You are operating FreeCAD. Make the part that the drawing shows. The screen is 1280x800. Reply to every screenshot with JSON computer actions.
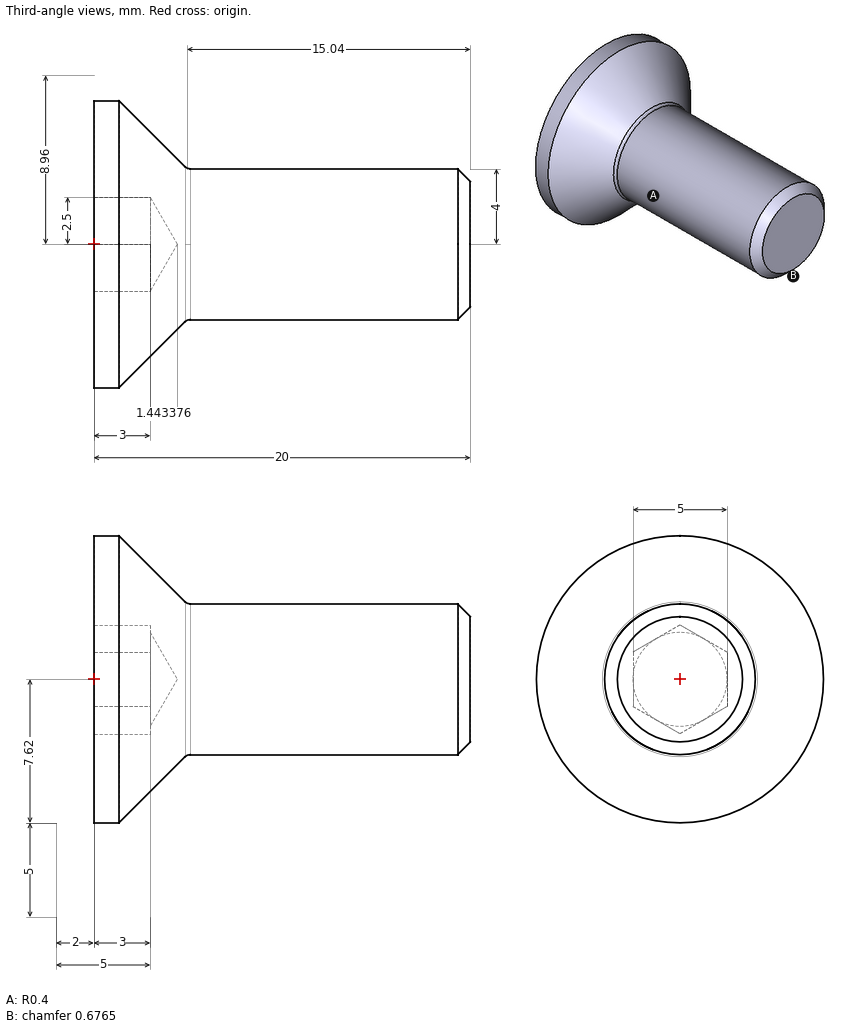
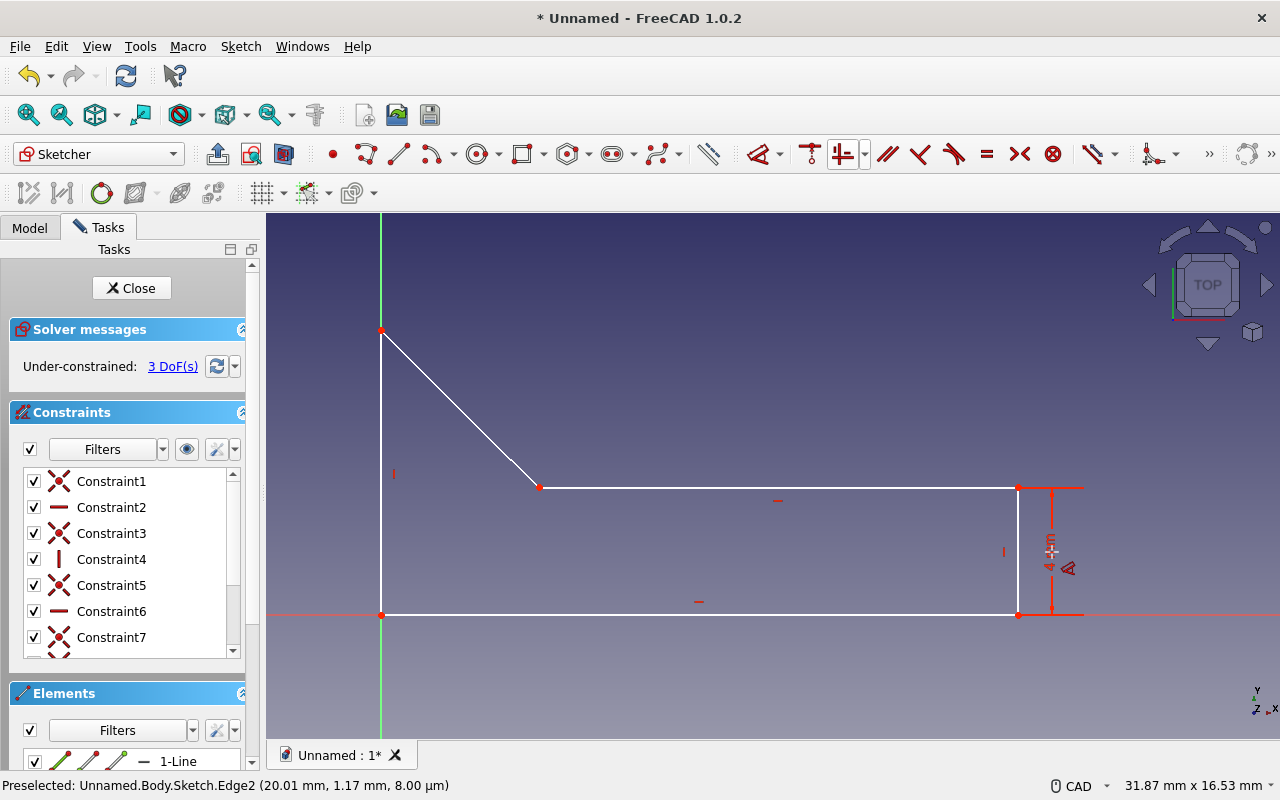
{"action": "left_click", "coordinate": [572, 615]}
{"action": "left_click", "coordinate": [700, 649]}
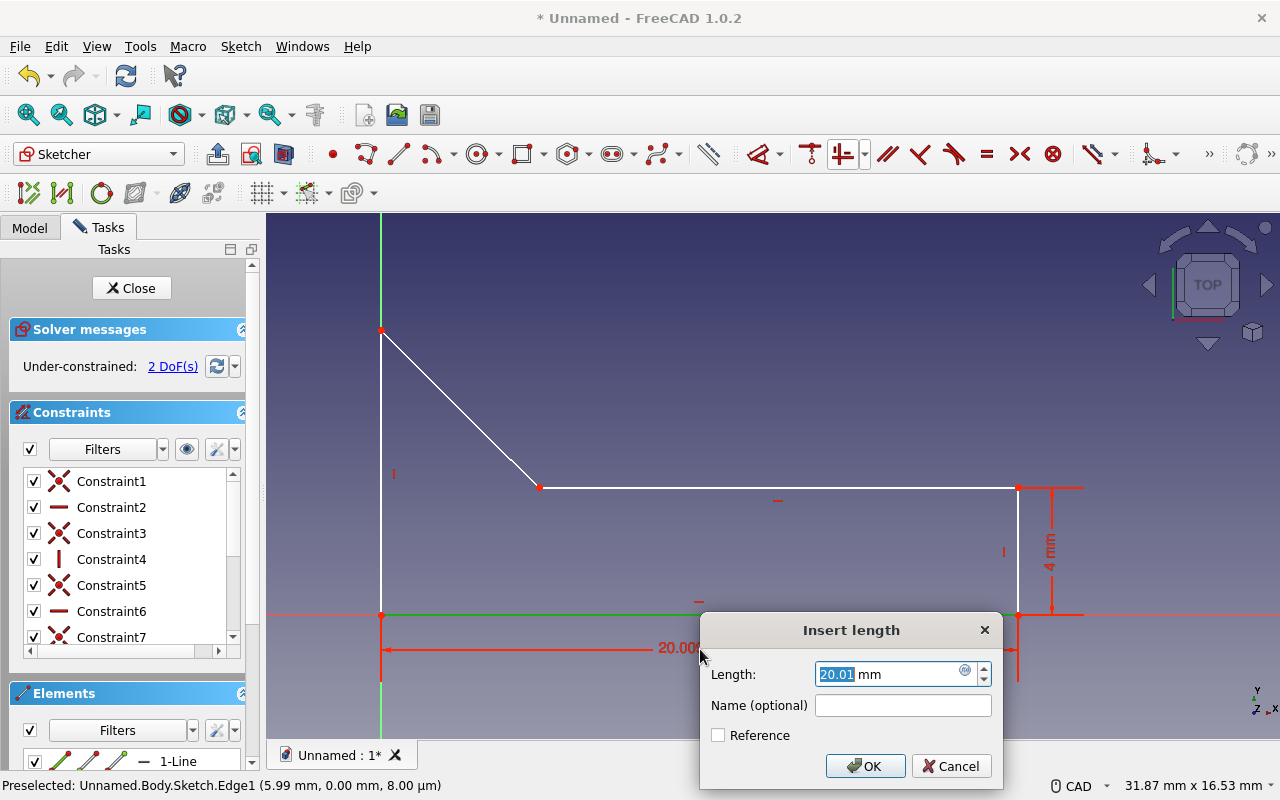
{"action": "type", "text": "20"}
{"action": "key", "text": "Return"}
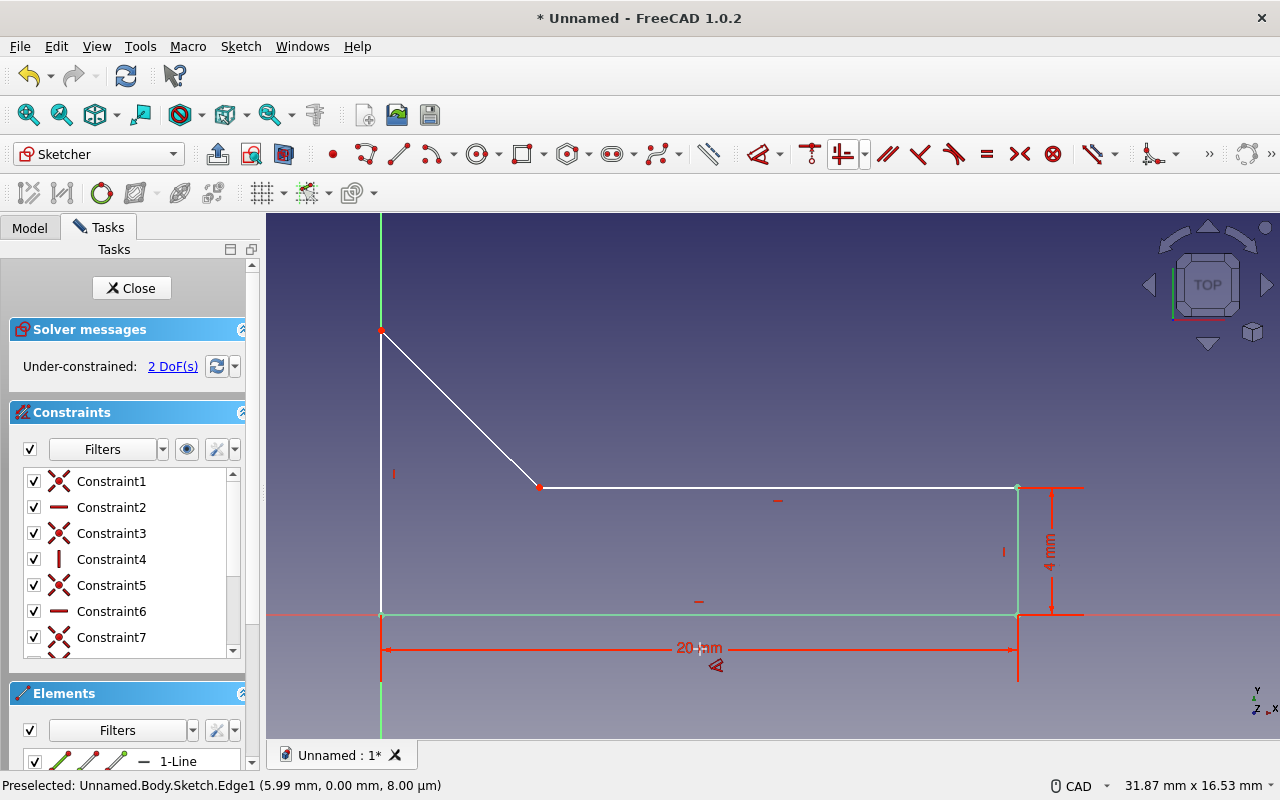
{"action": "left_click", "coordinate": [381, 416]}
{"action": "left_click", "coordinate": [347, 473]}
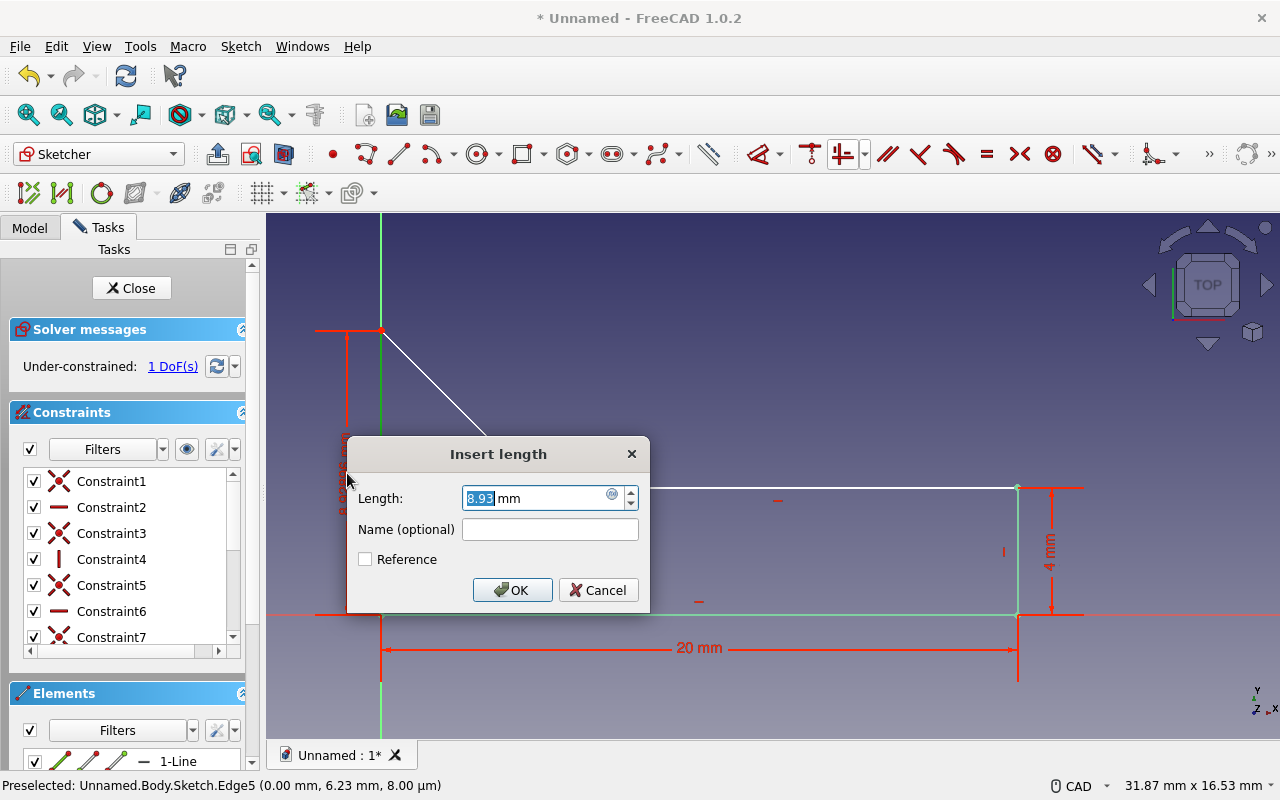
{"action": "type", "text": "8.96"}
{"action": "key", "text": "Return"}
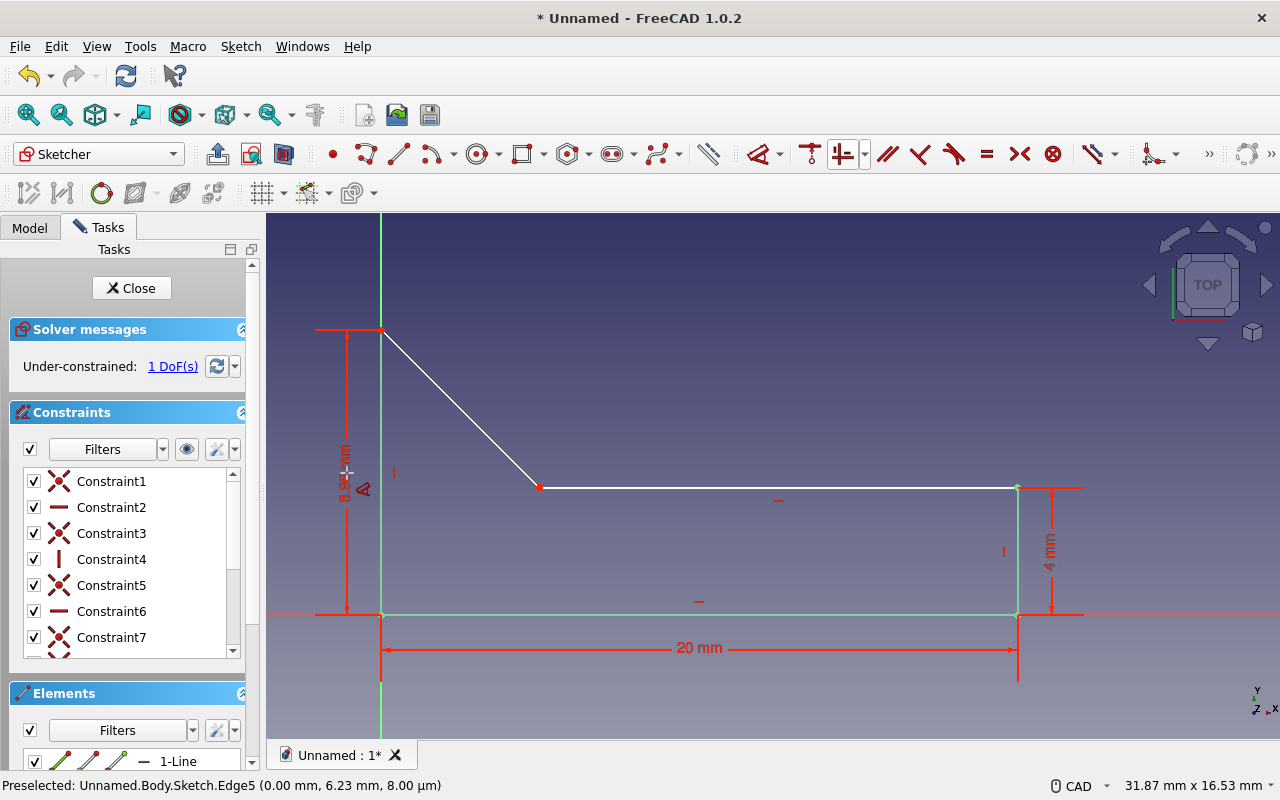
{"action": "left_click", "coordinate": [874, 488]}
{"action": "left_click", "coordinate": [778, 522]}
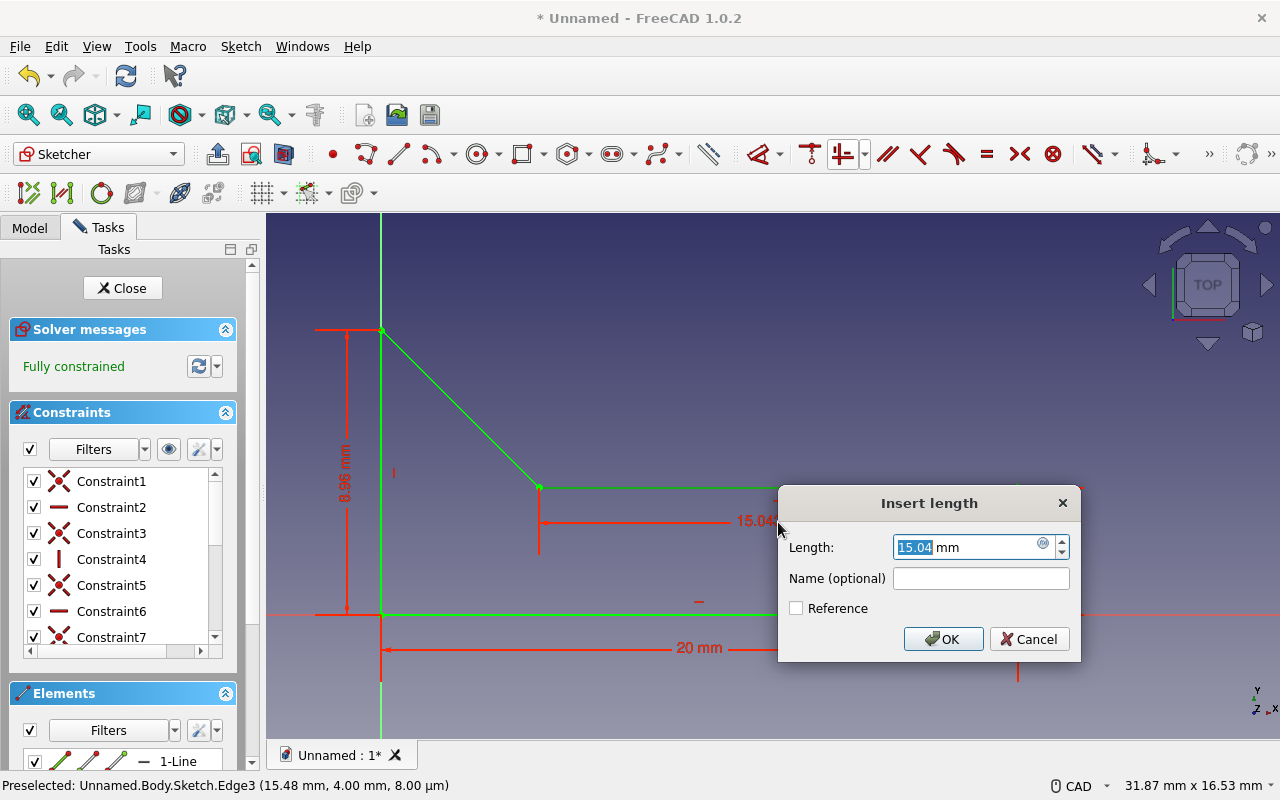
{"action": "type", "text": "15.04"}
{"action": "key", "text": "Return"}
{"action": "key", "text": "Escape"}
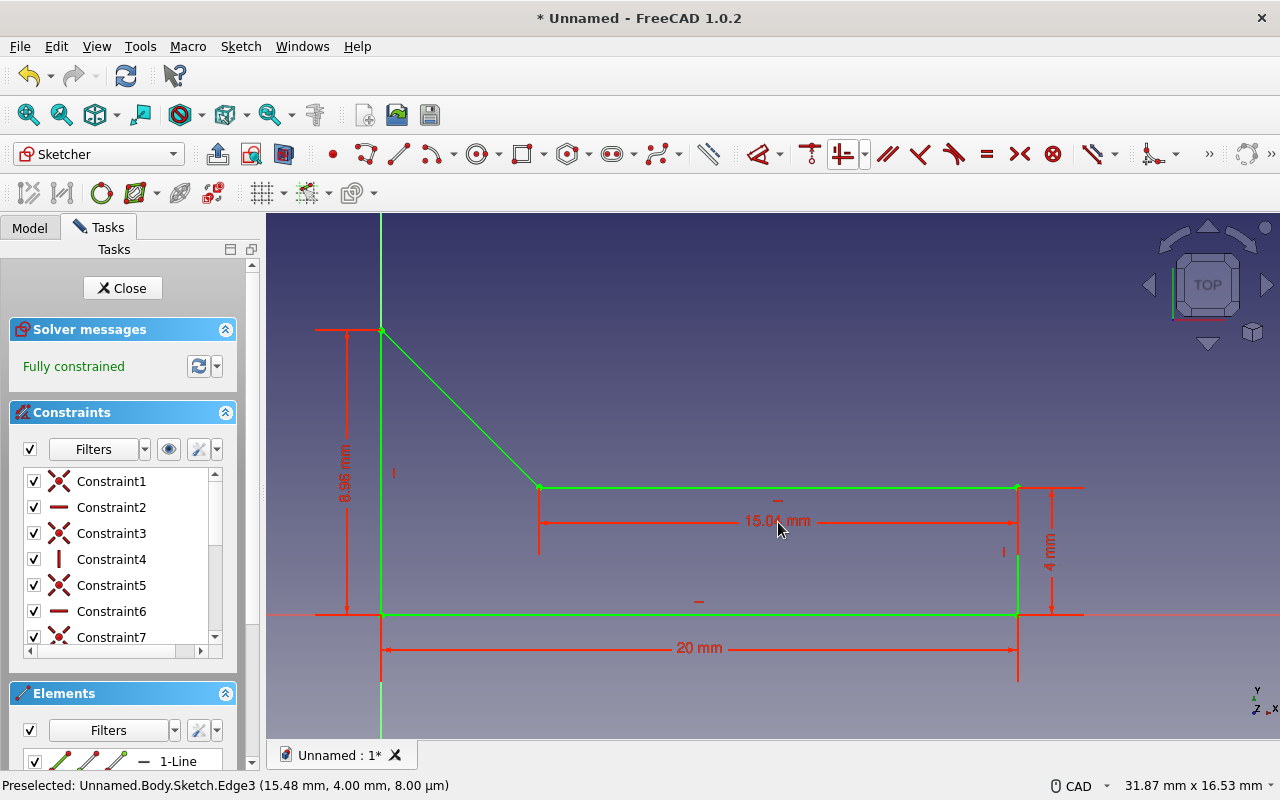
{"action": "left_click", "coordinate": [123, 288]}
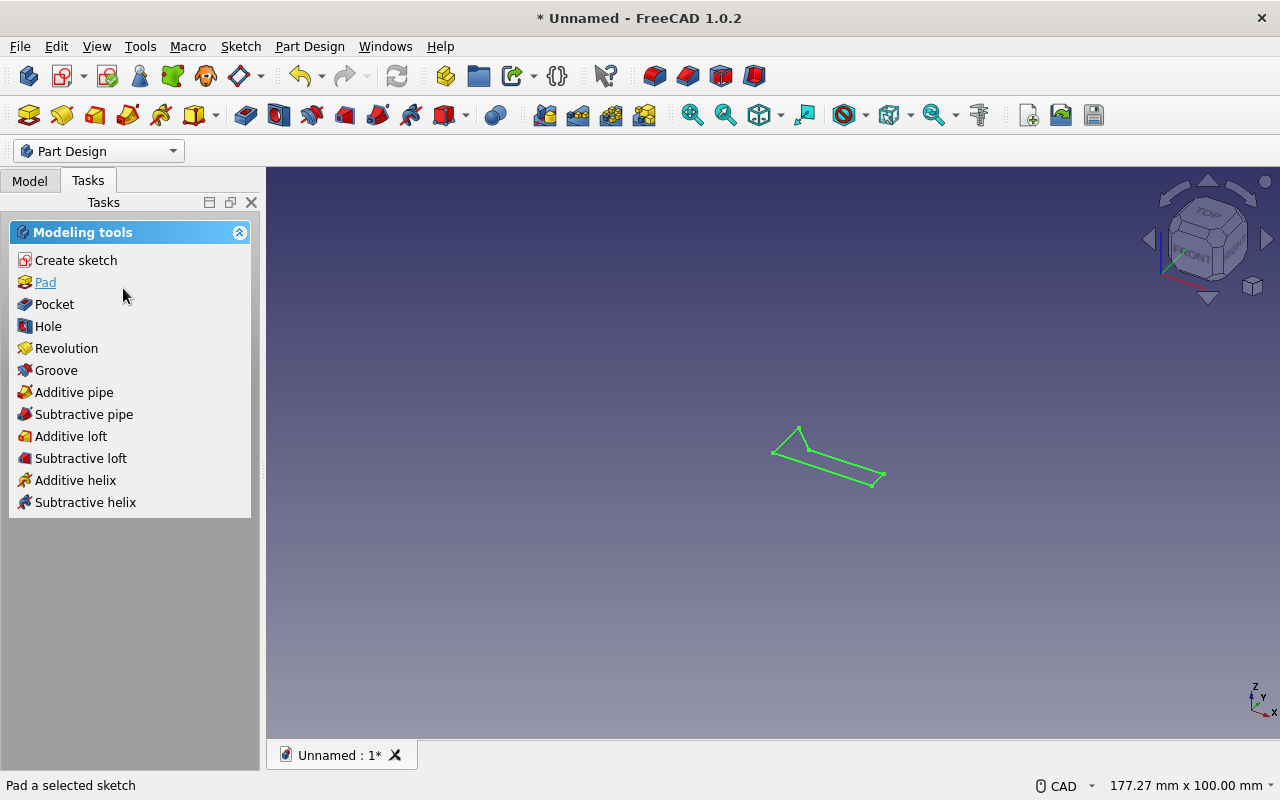
{"action": "left_click", "coordinate": [62, 116]}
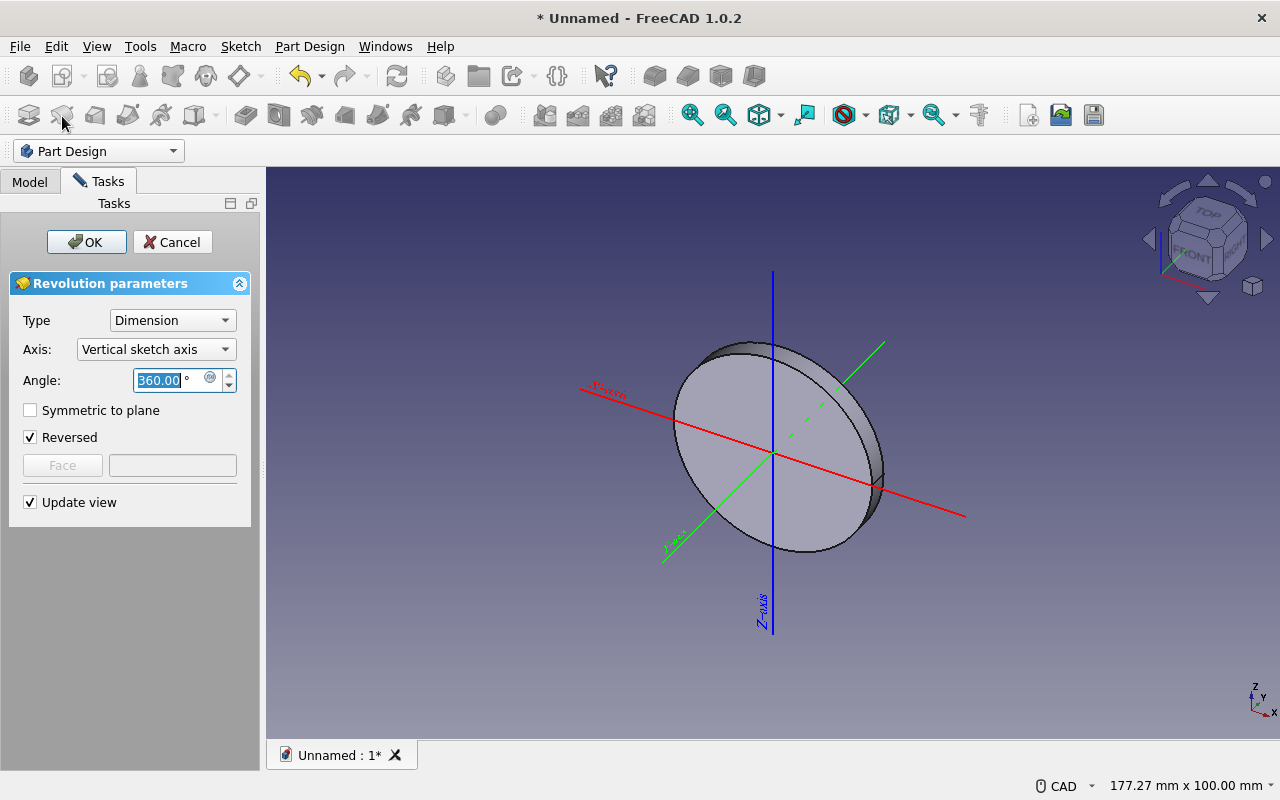
{"action": "left_click", "coordinate": [157, 350]}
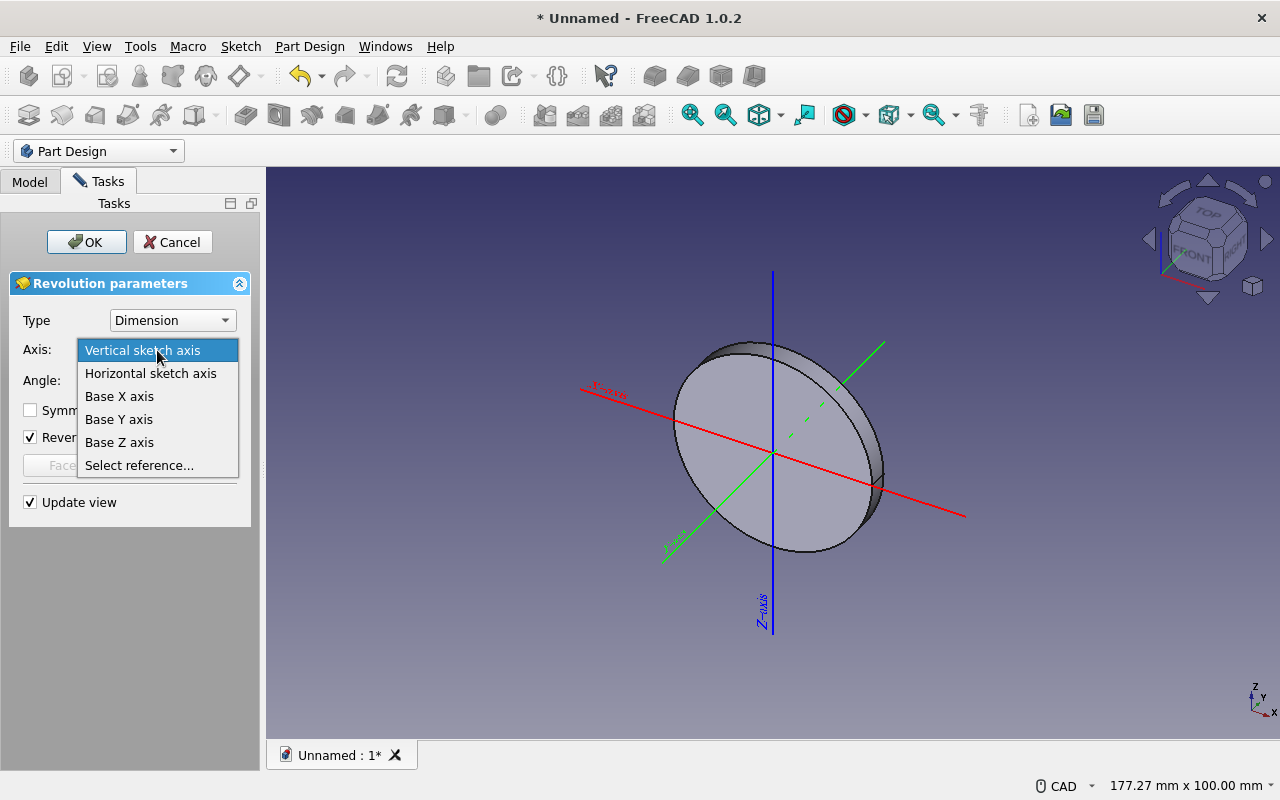
{"action": "left_click", "coordinate": [156, 374]}